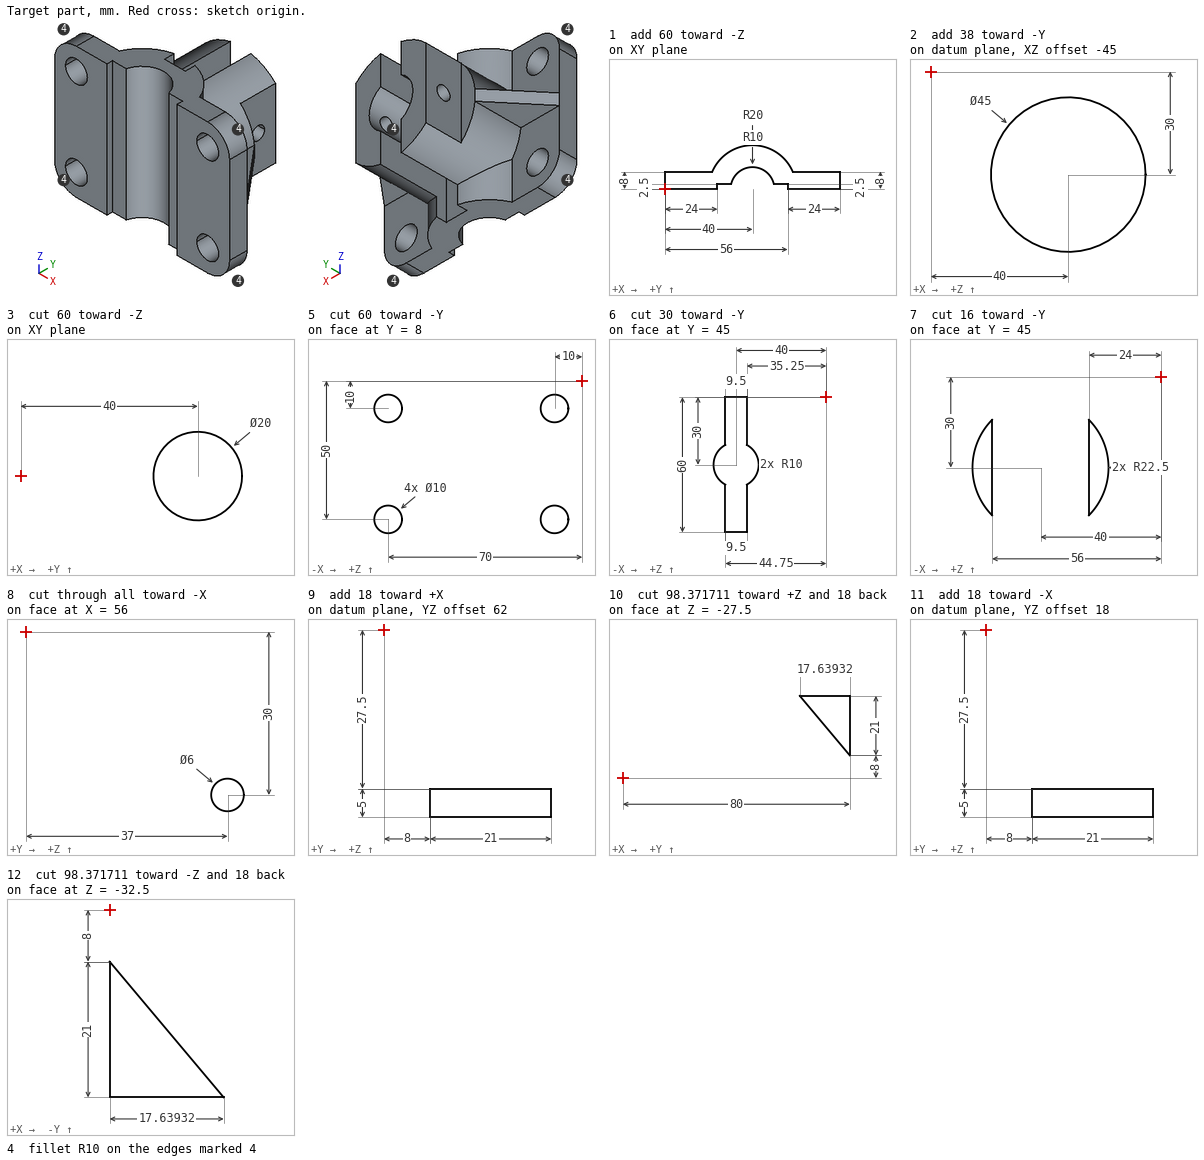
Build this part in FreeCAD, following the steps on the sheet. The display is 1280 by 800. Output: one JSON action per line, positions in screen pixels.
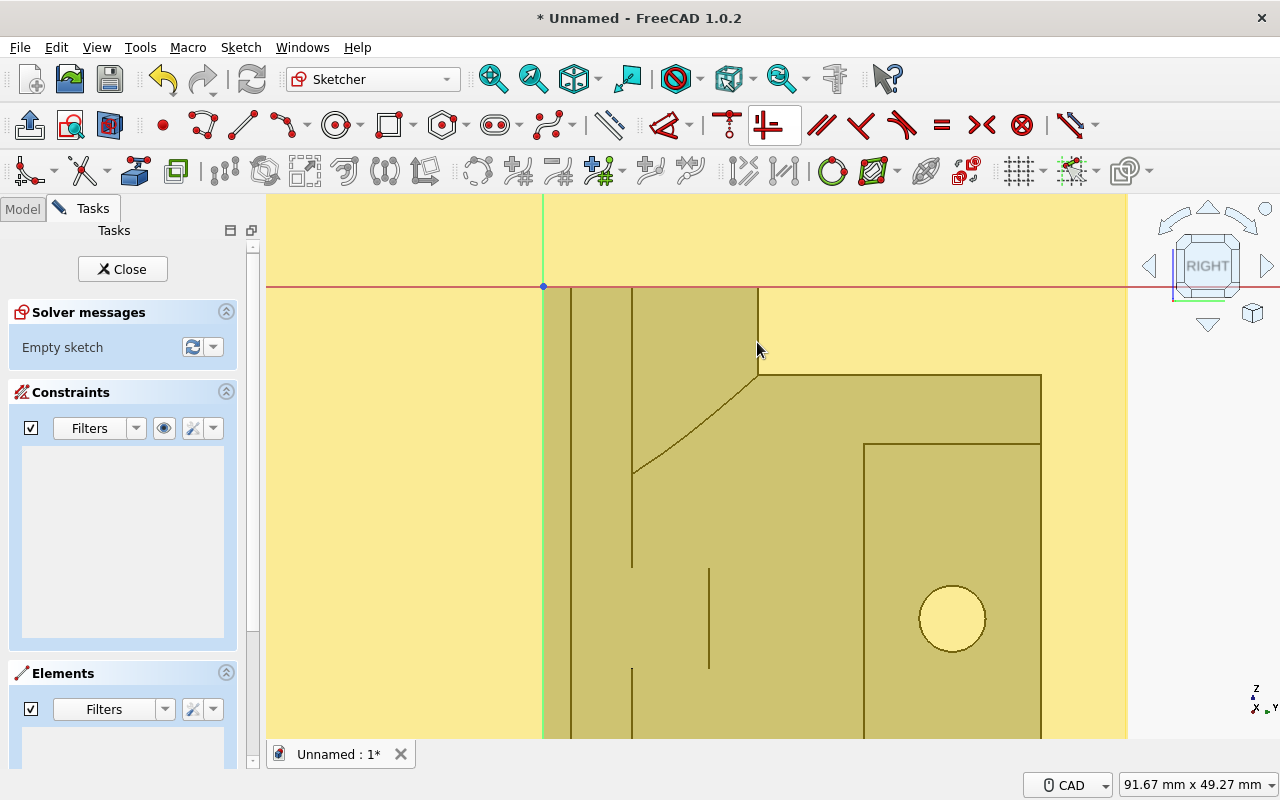
{"action": "left_click", "coordinate": [390, 126]}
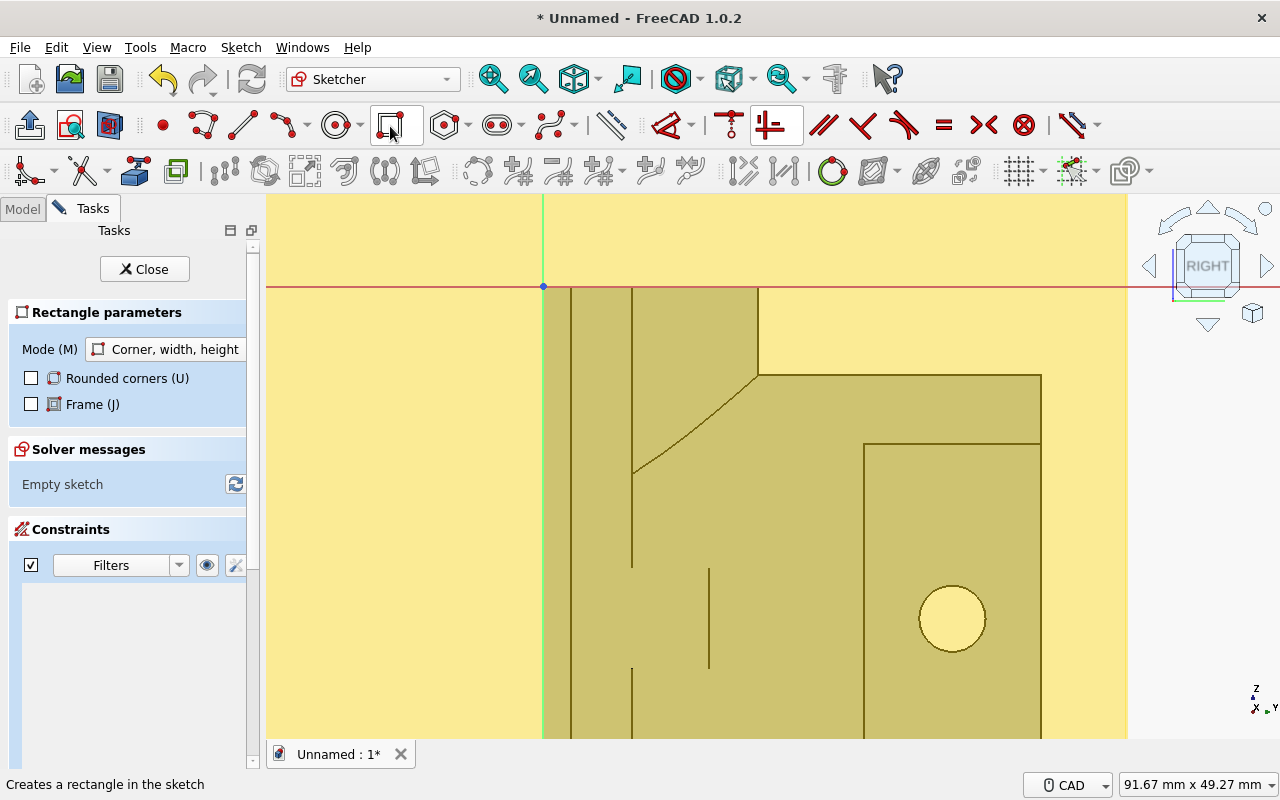
{"action": "left_click", "coordinate": [632, 591]}
{"action": "left_click", "coordinate": [864, 646]}
{"action": "key", "text": "Escape"}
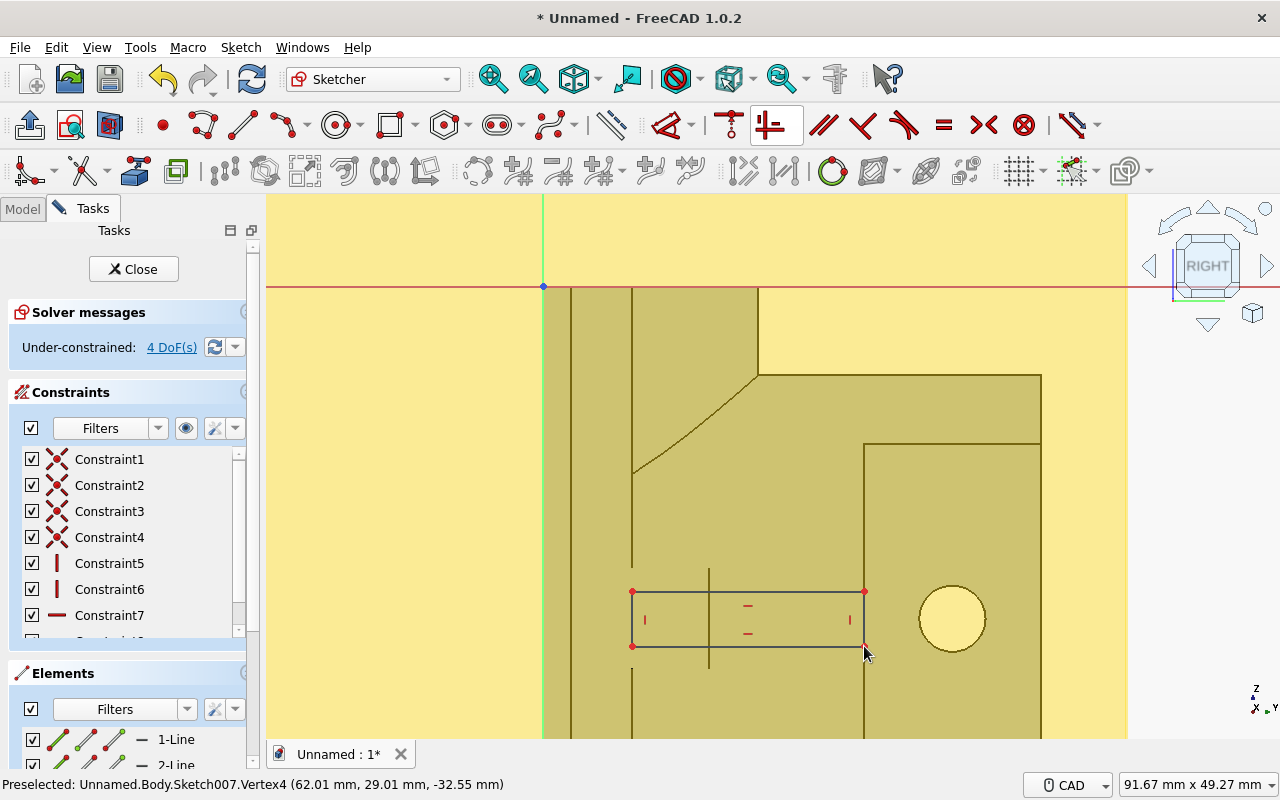
{"action": "left_click", "coordinate": [666, 126]}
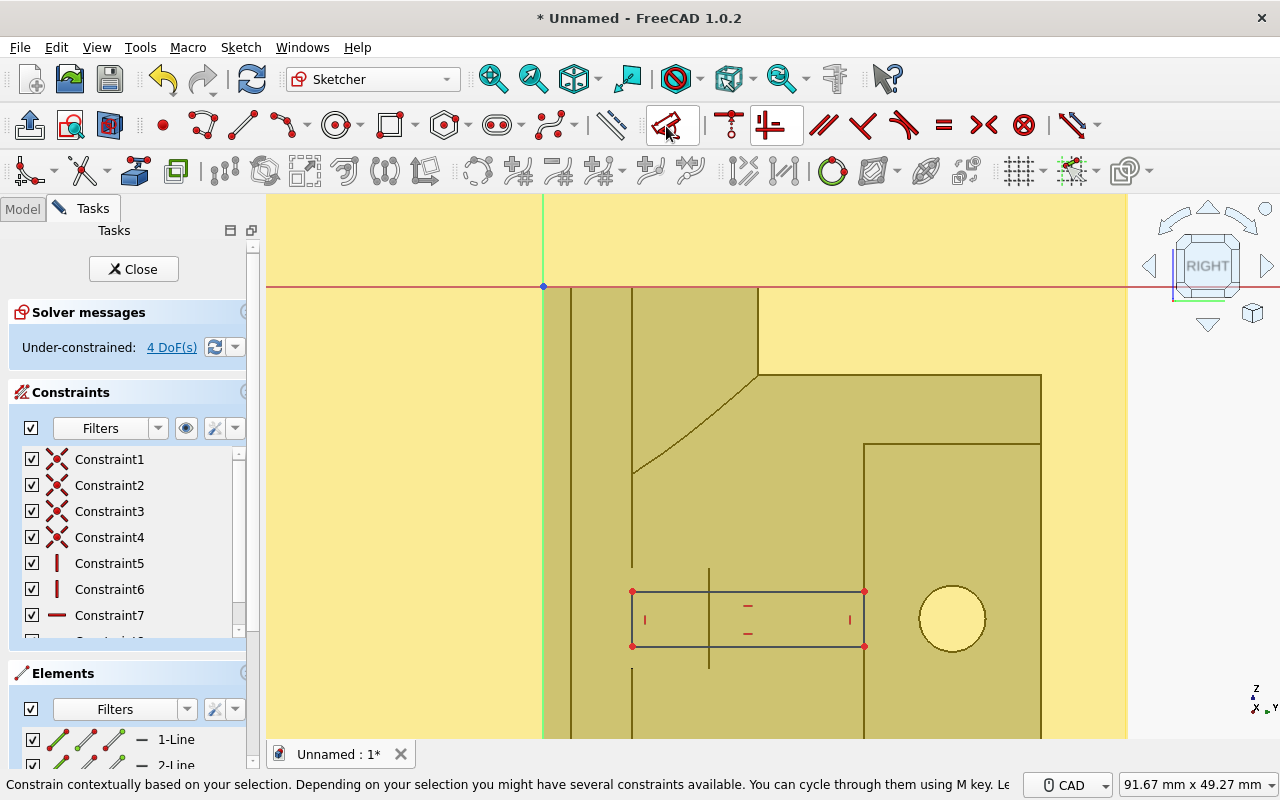
{"action": "left_click", "coordinate": [632, 608]}
{"action": "left_click", "coordinate": [598, 619]}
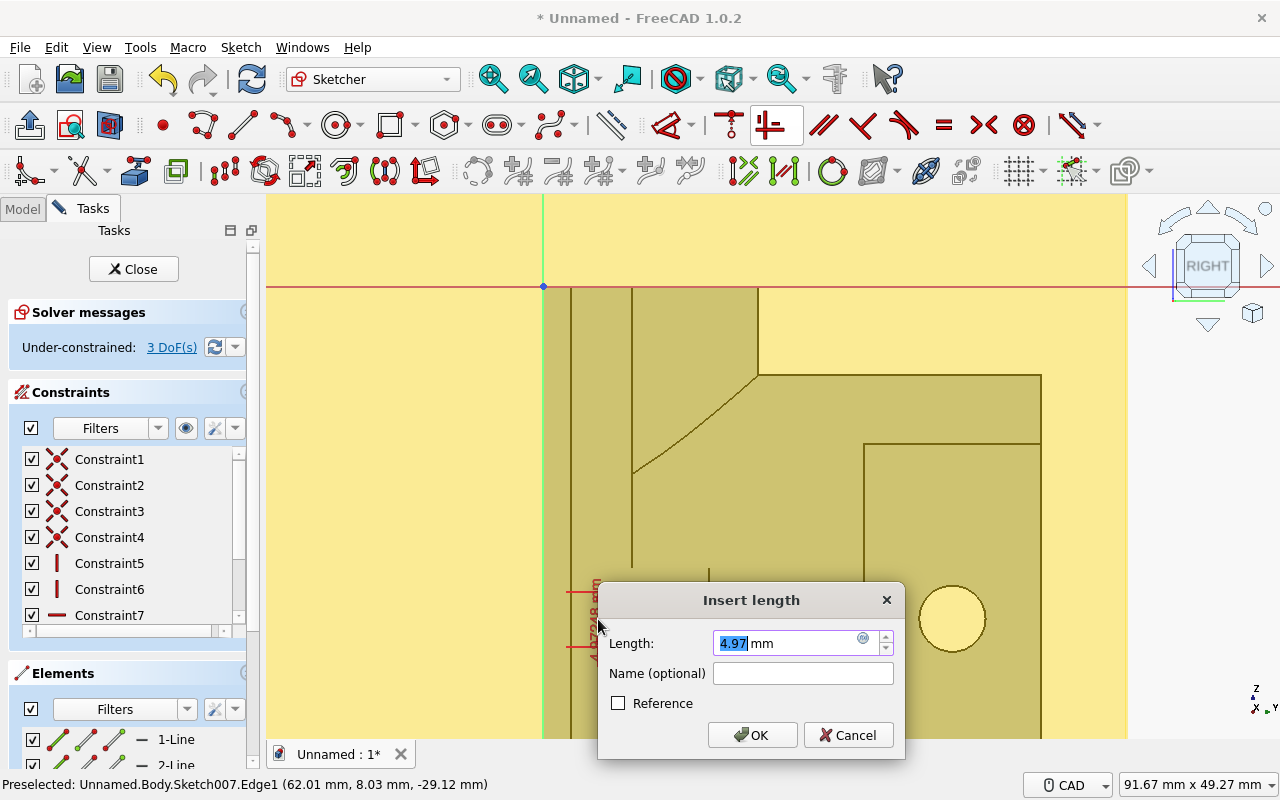
{"action": "type", "text": "5"}
{"action": "key", "text": "Return"}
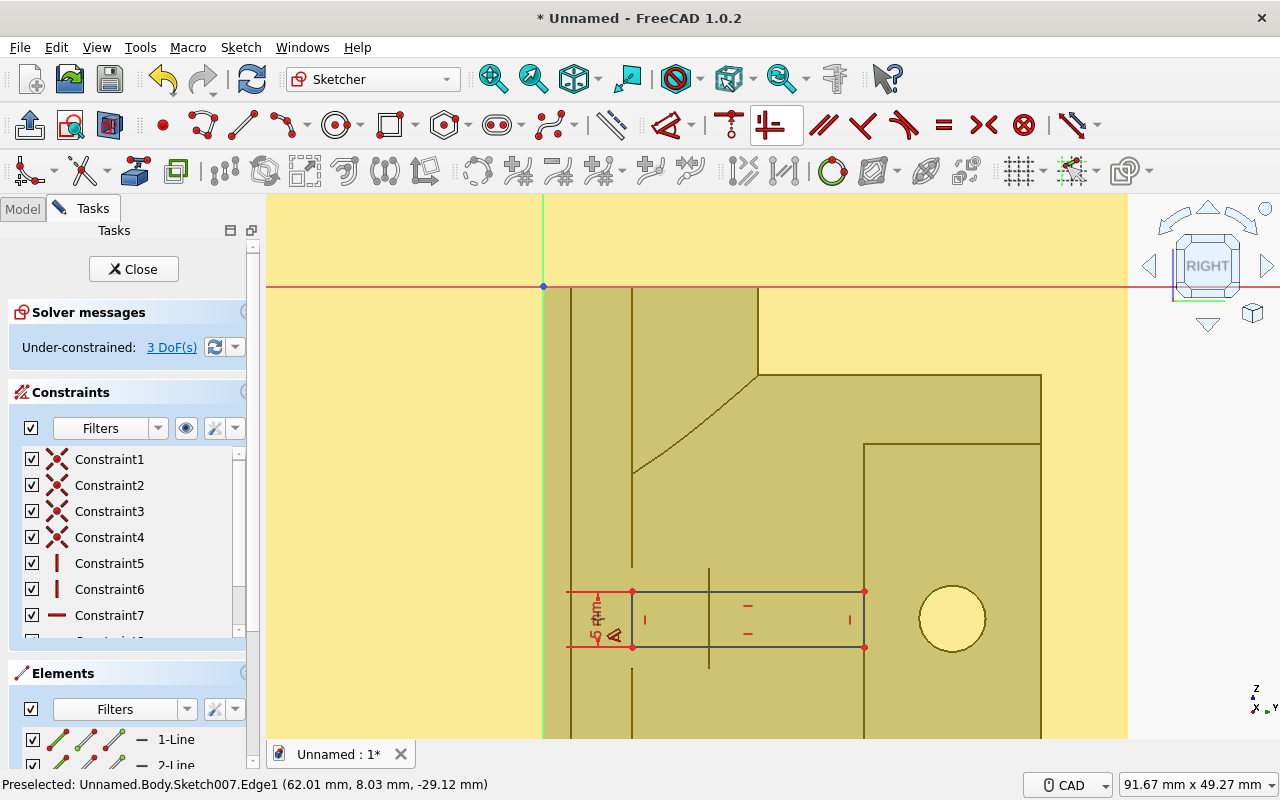
{"action": "left_click", "coordinate": [702, 647]}
{"action": "left_click", "coordinate": [748, 681]}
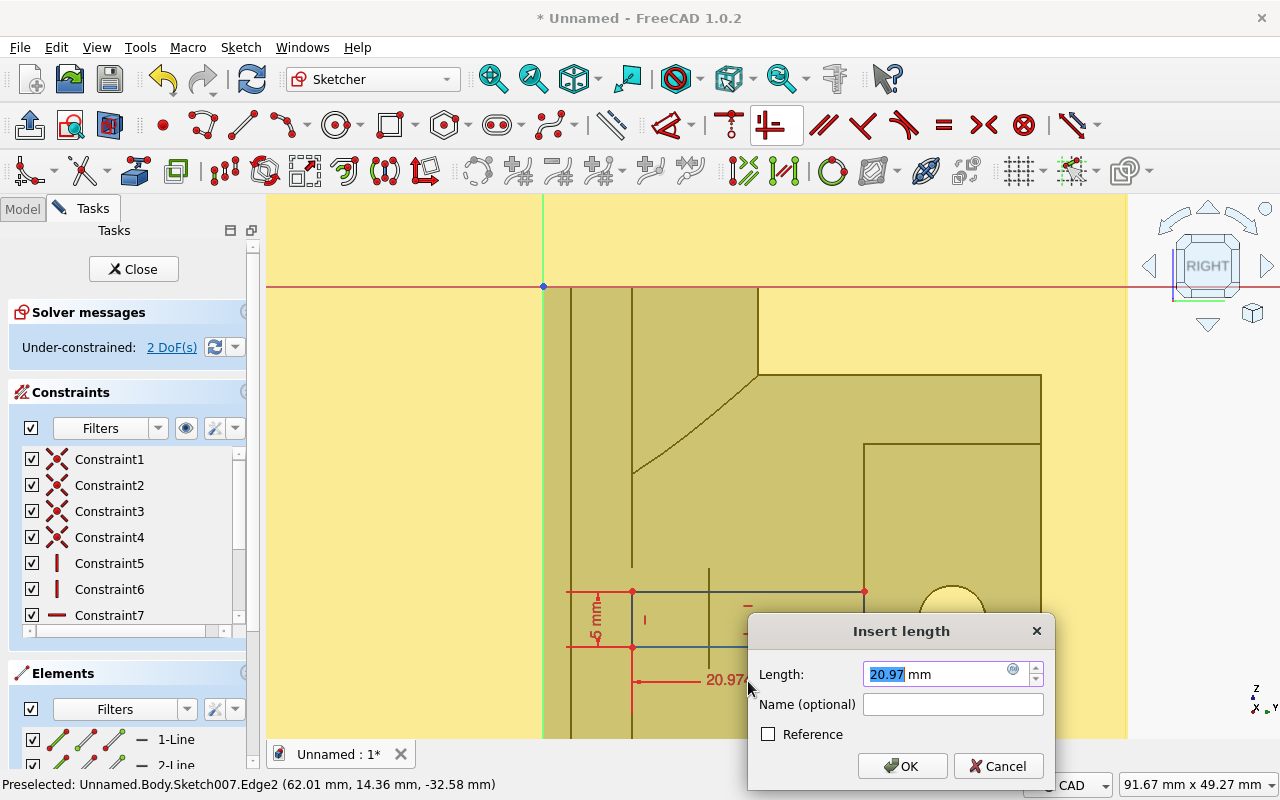
{"action": "type", "text": "21"}
{"action": "key", "text": "Return"}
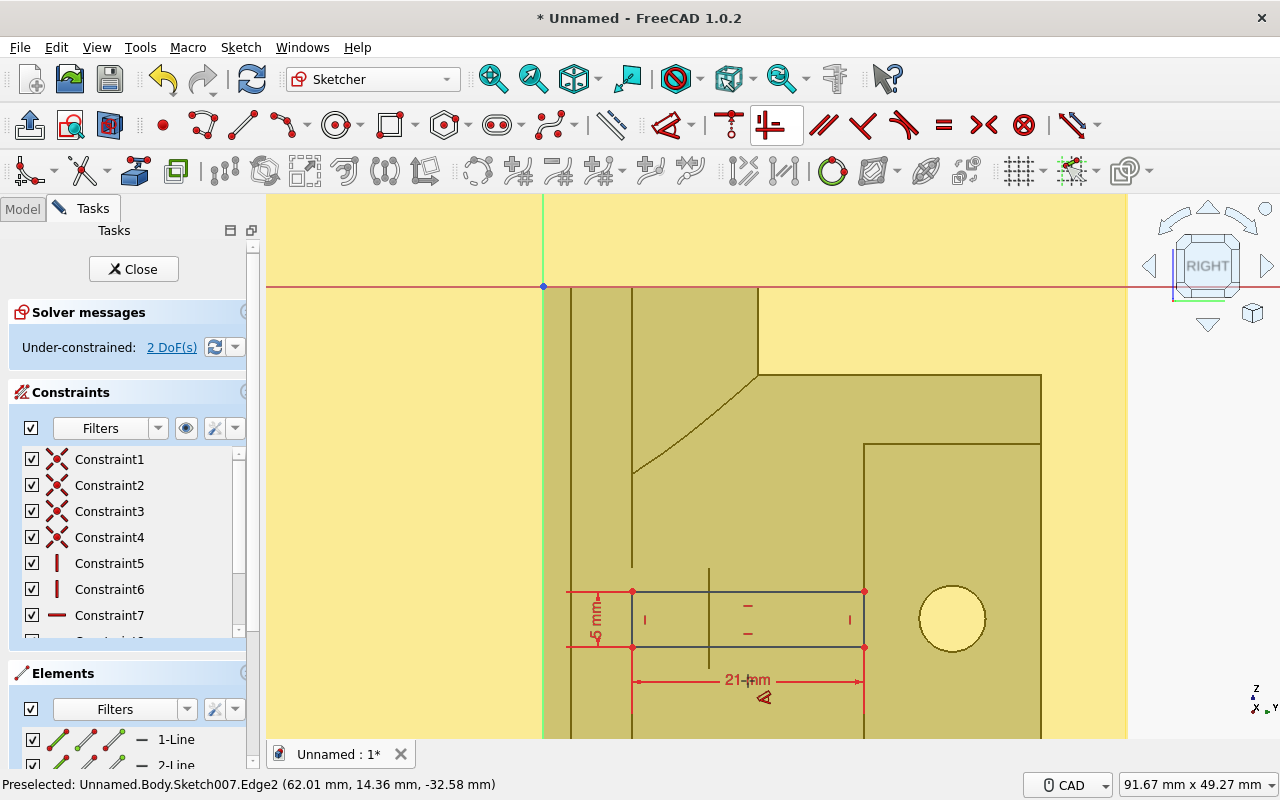
{"action": "left_click", "coordinate": [632, 592]}
{"action": "left_click", "coordinate": [588, 253]}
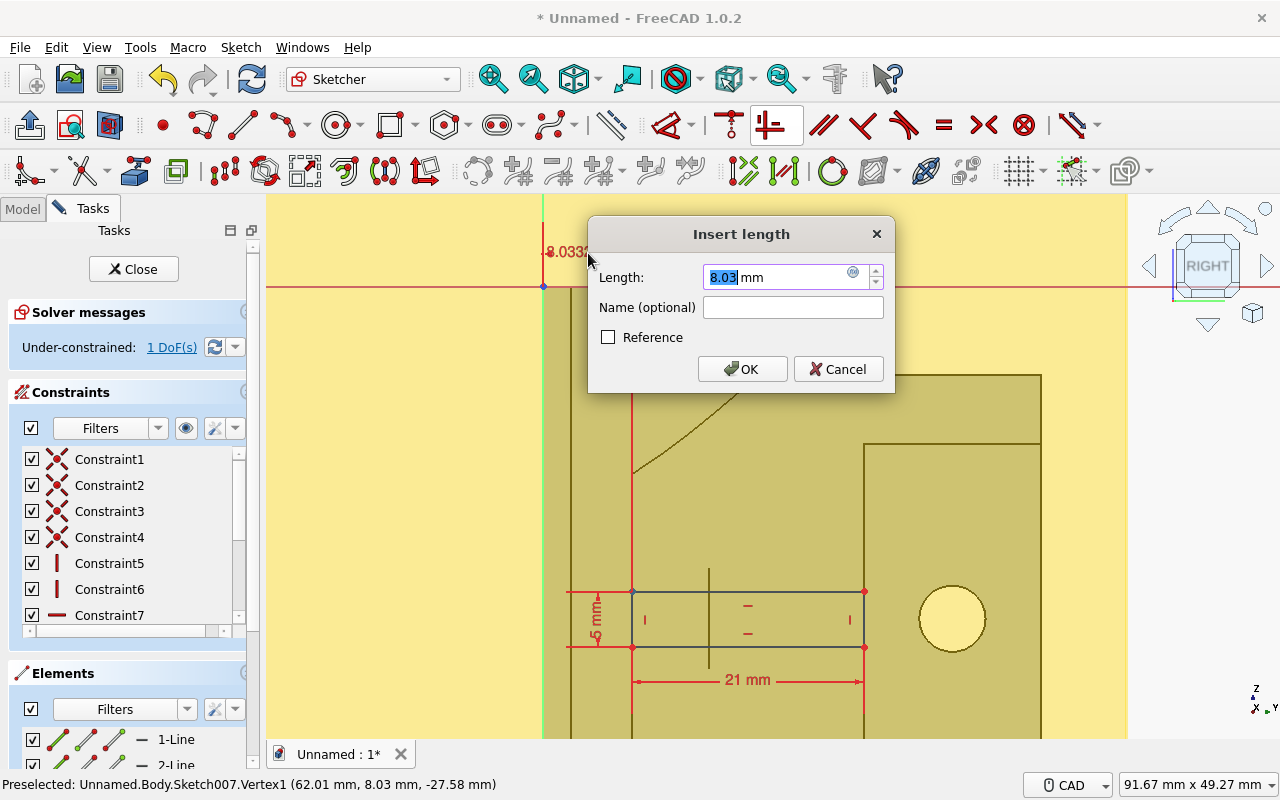
{"action": "type", "text": "8"}
{"action": "key", "text": "Return"}